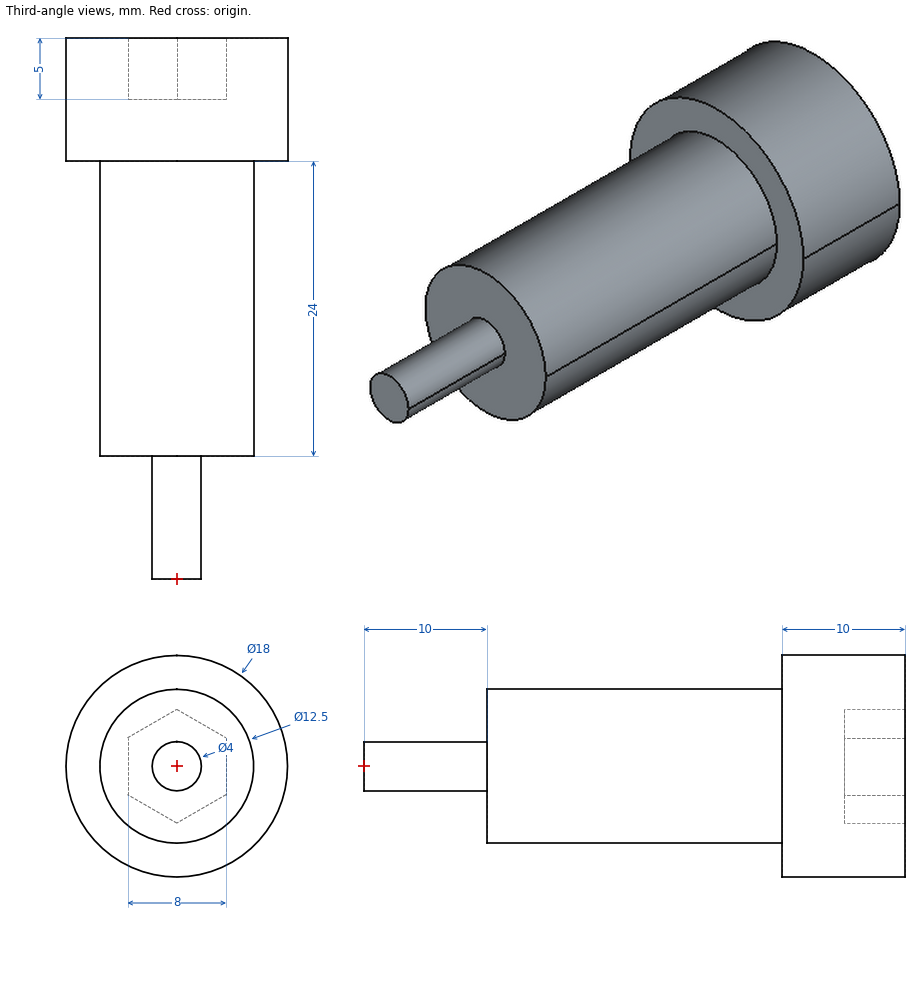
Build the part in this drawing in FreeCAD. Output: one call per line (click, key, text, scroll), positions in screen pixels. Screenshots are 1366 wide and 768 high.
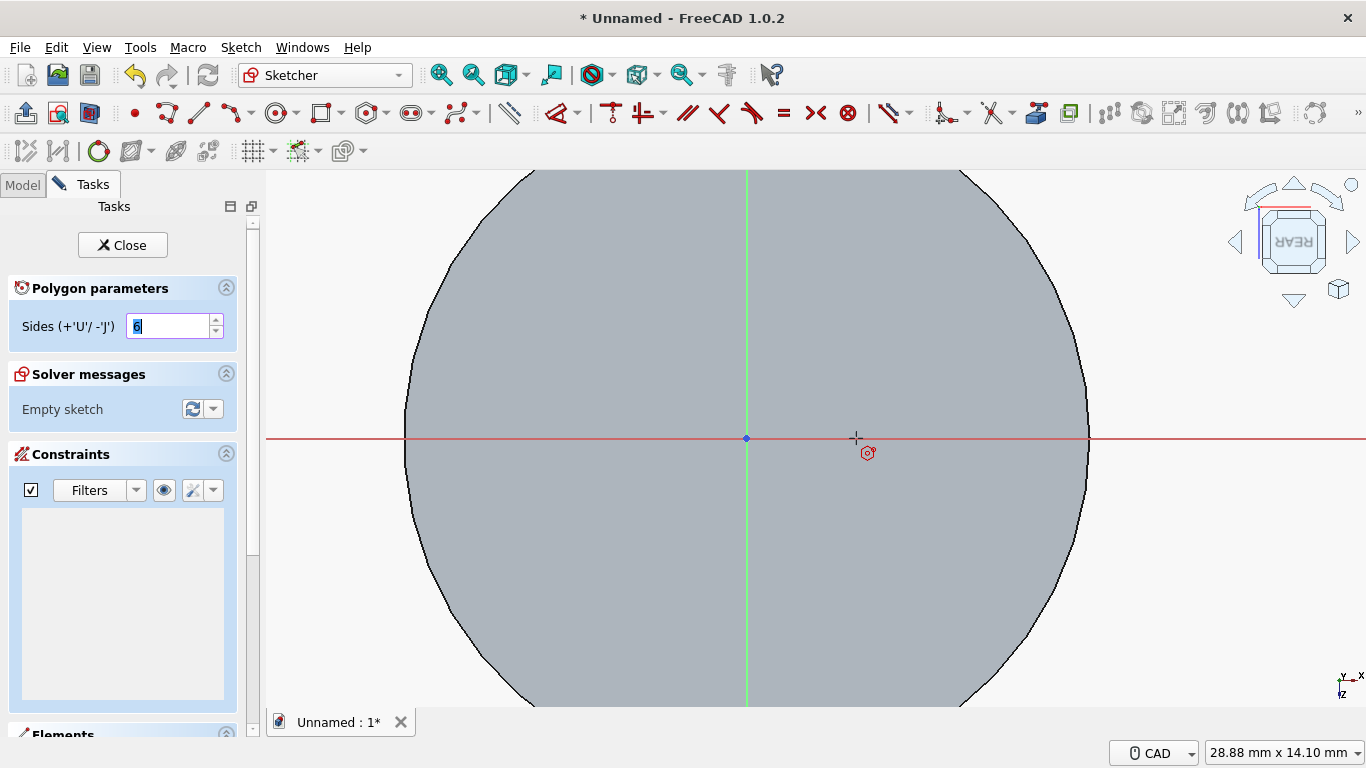
click(747, 438)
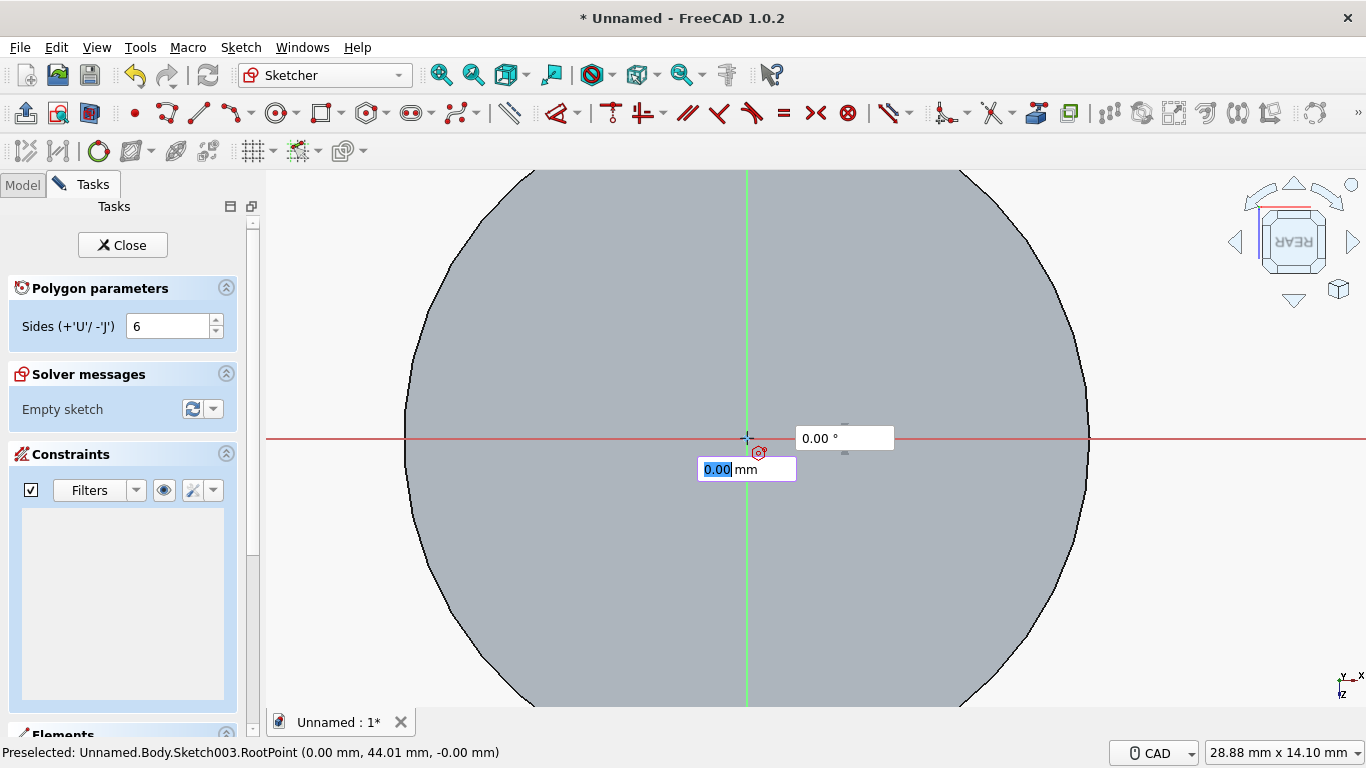
click(747, 263)
right_click(747, 263)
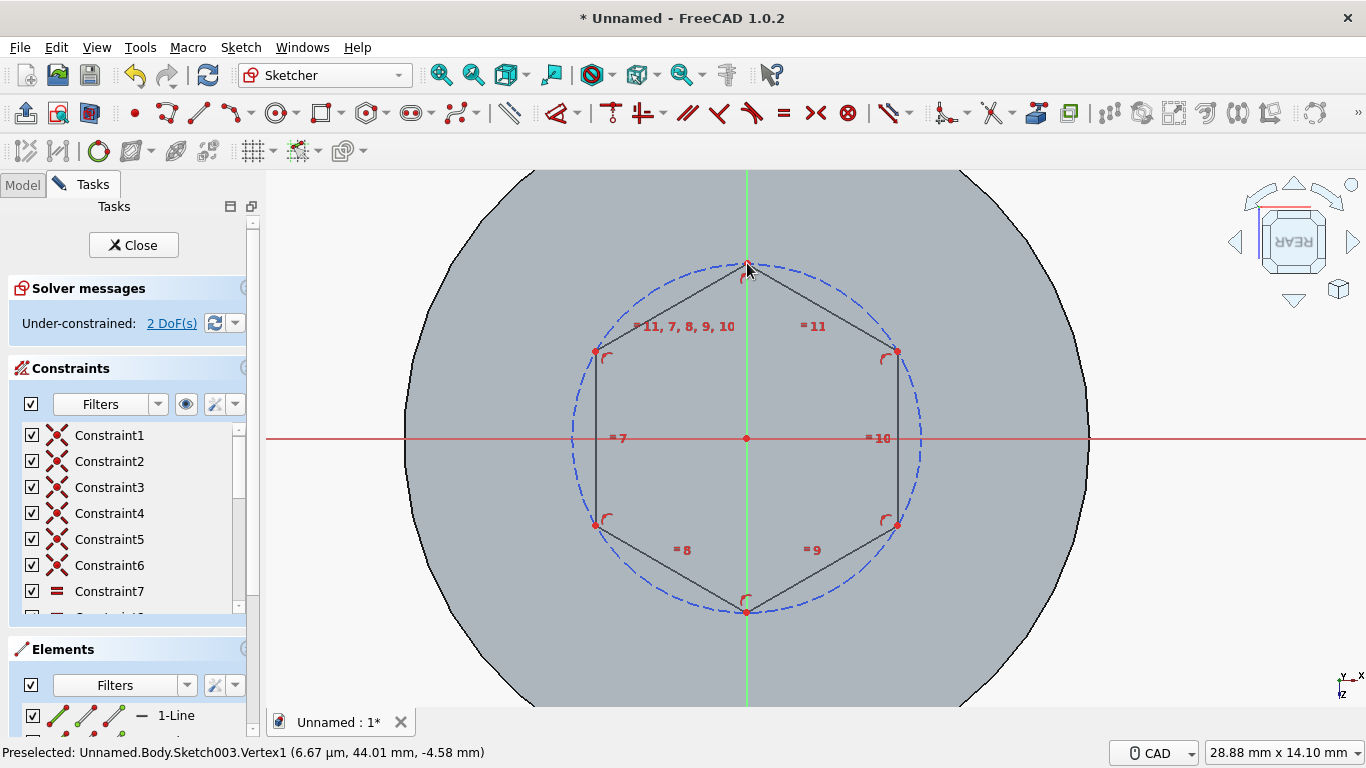
click(596, 403)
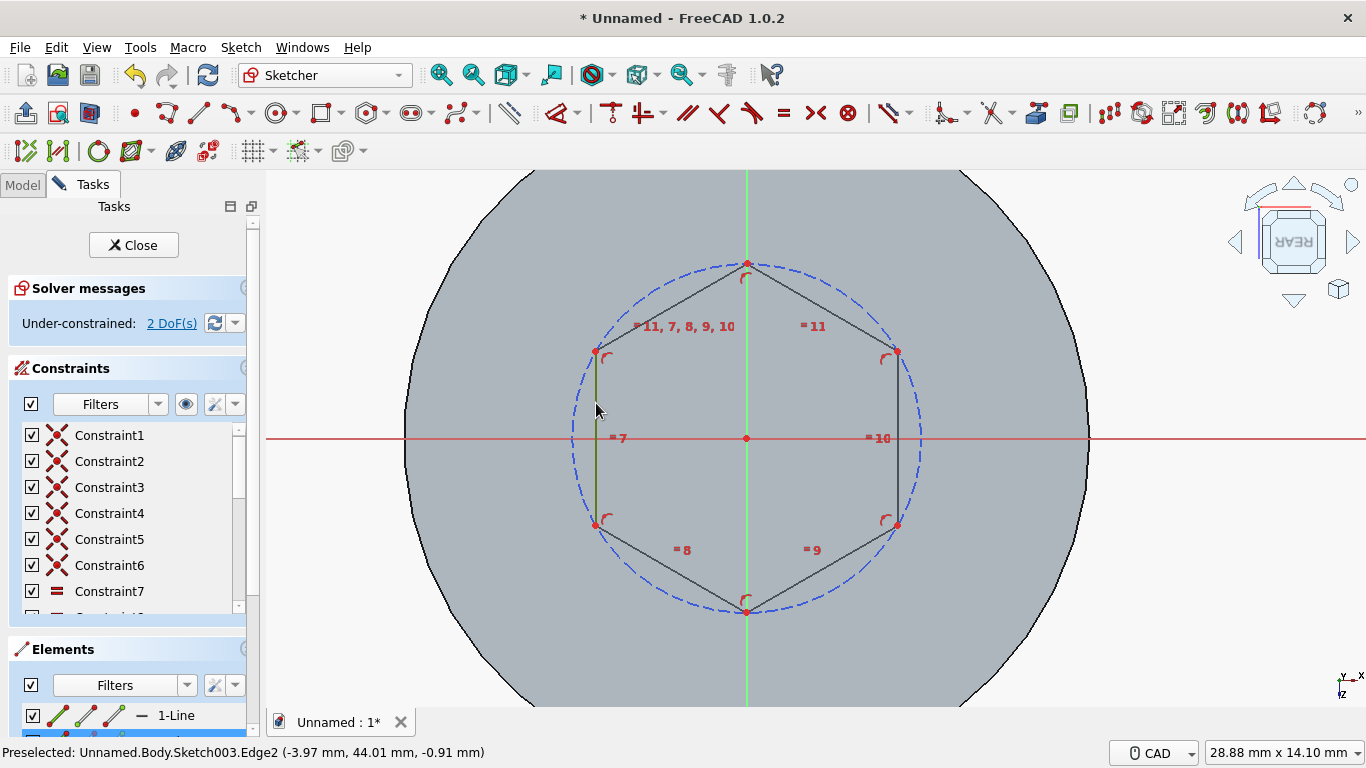
key(v)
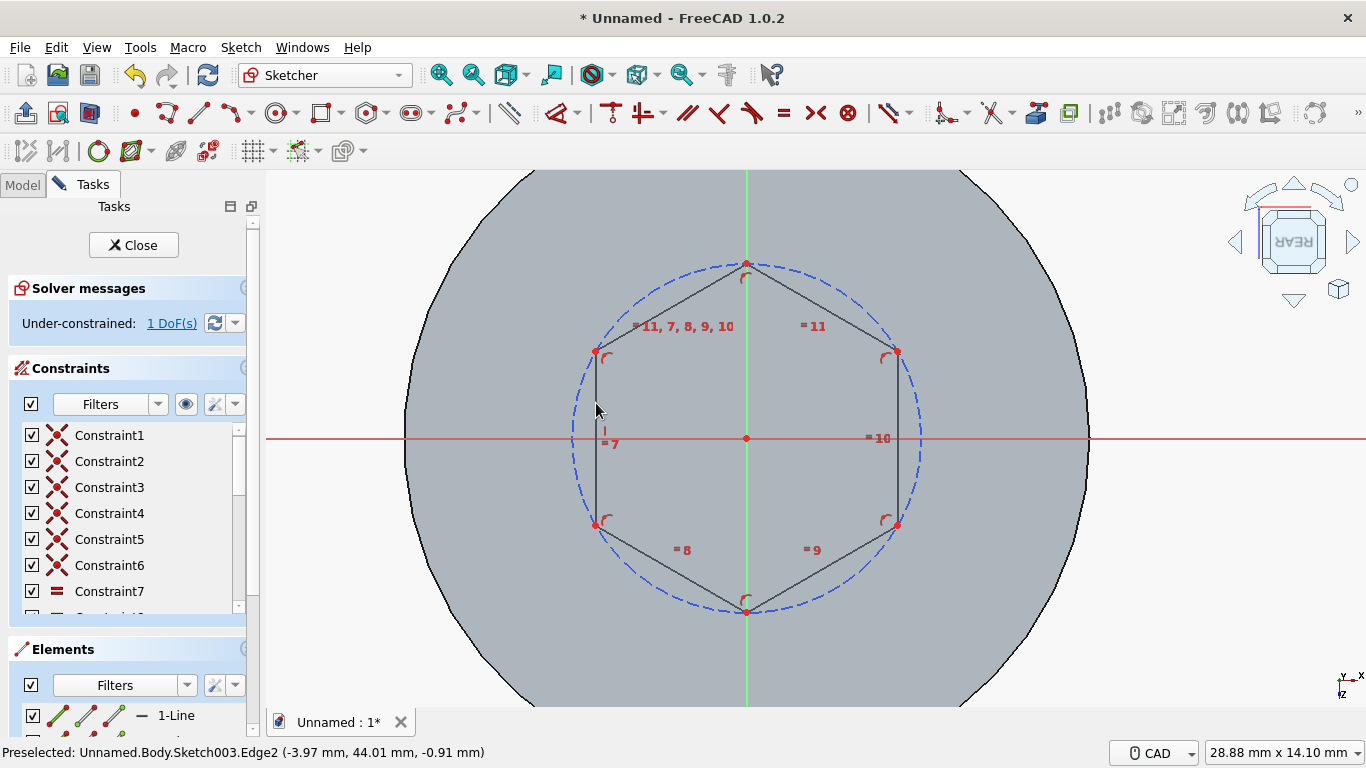
key(d)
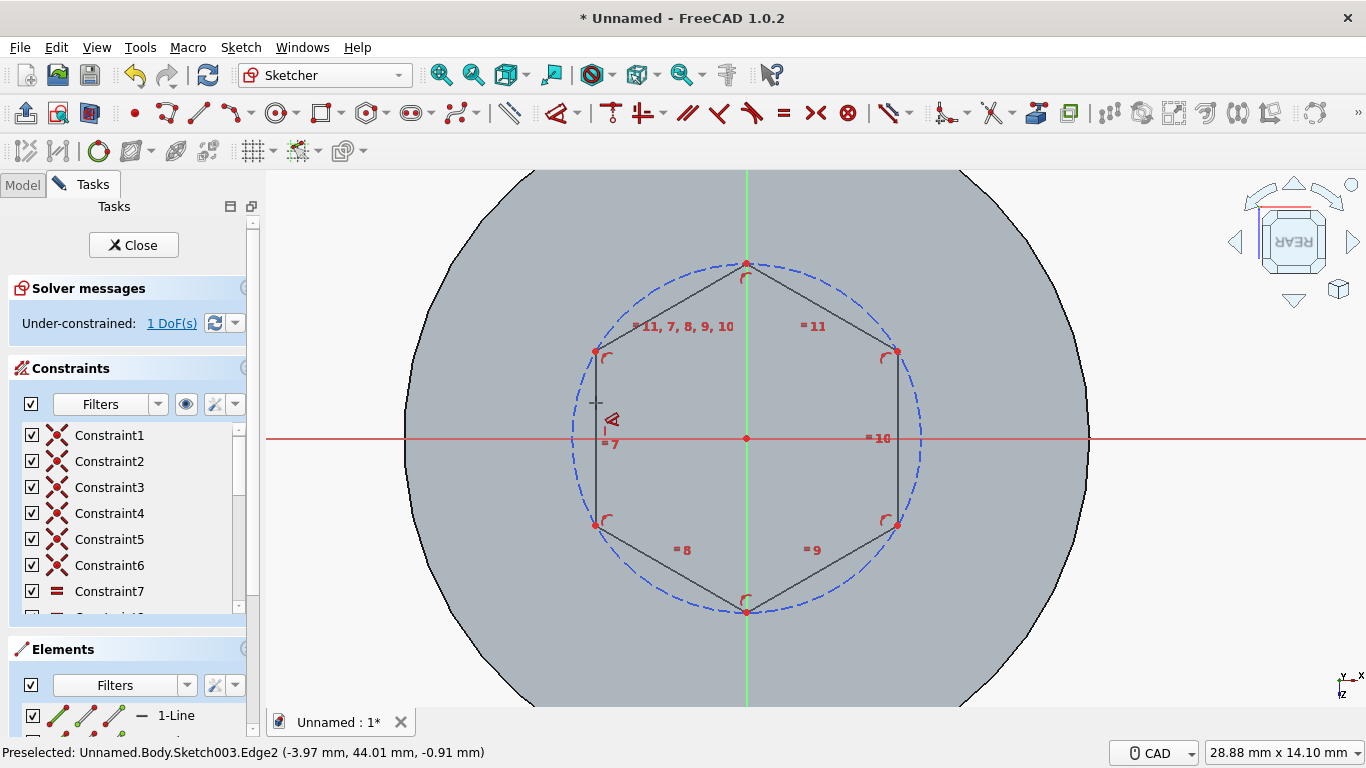
click(596, 351)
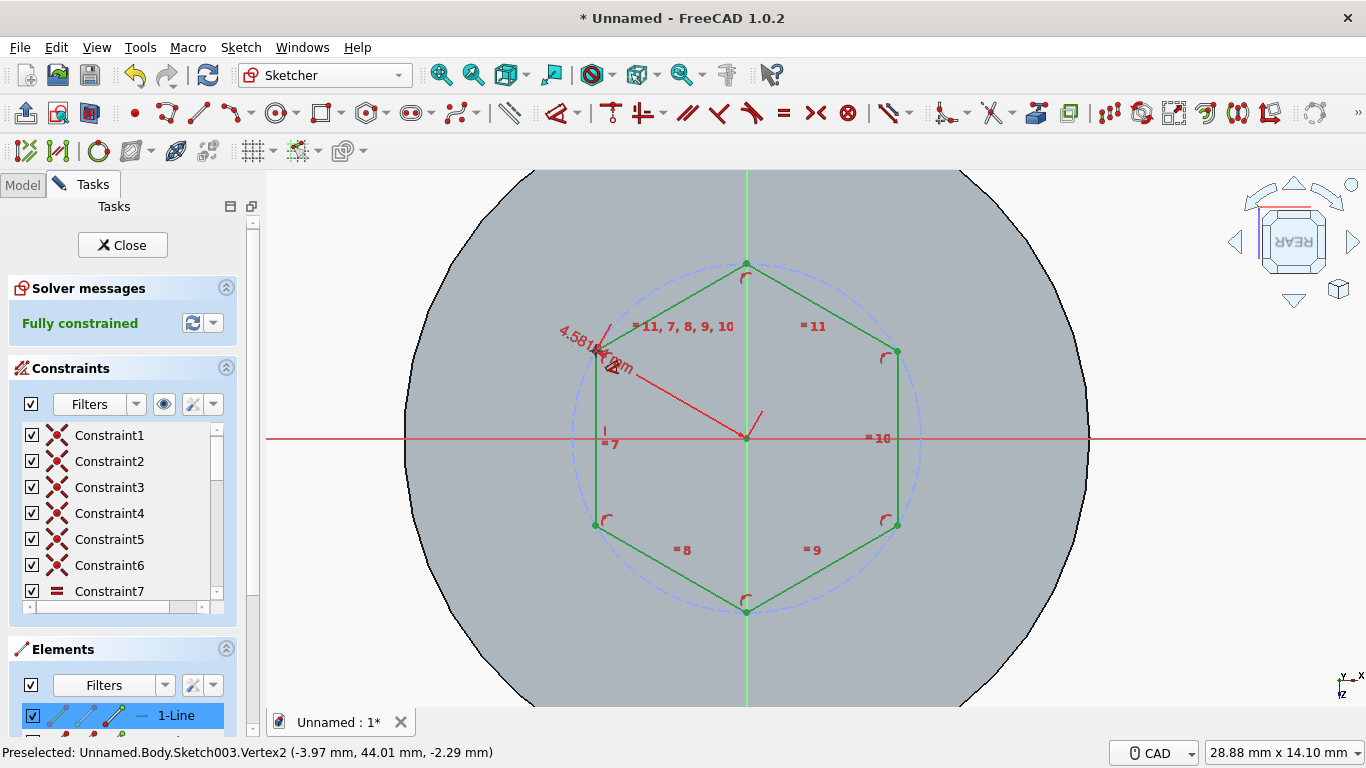
click(898, 526)
click(641, 269)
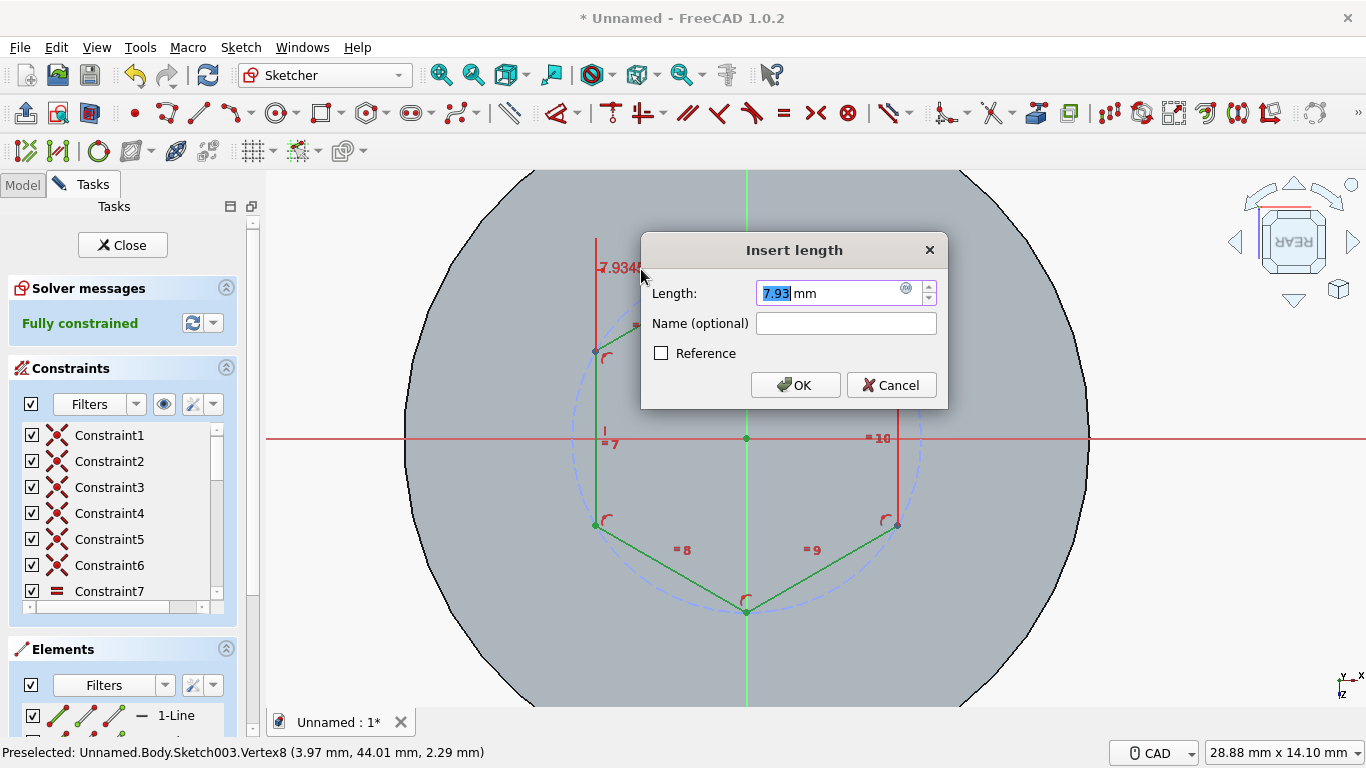
text(8)
key(Return)
key(Escape)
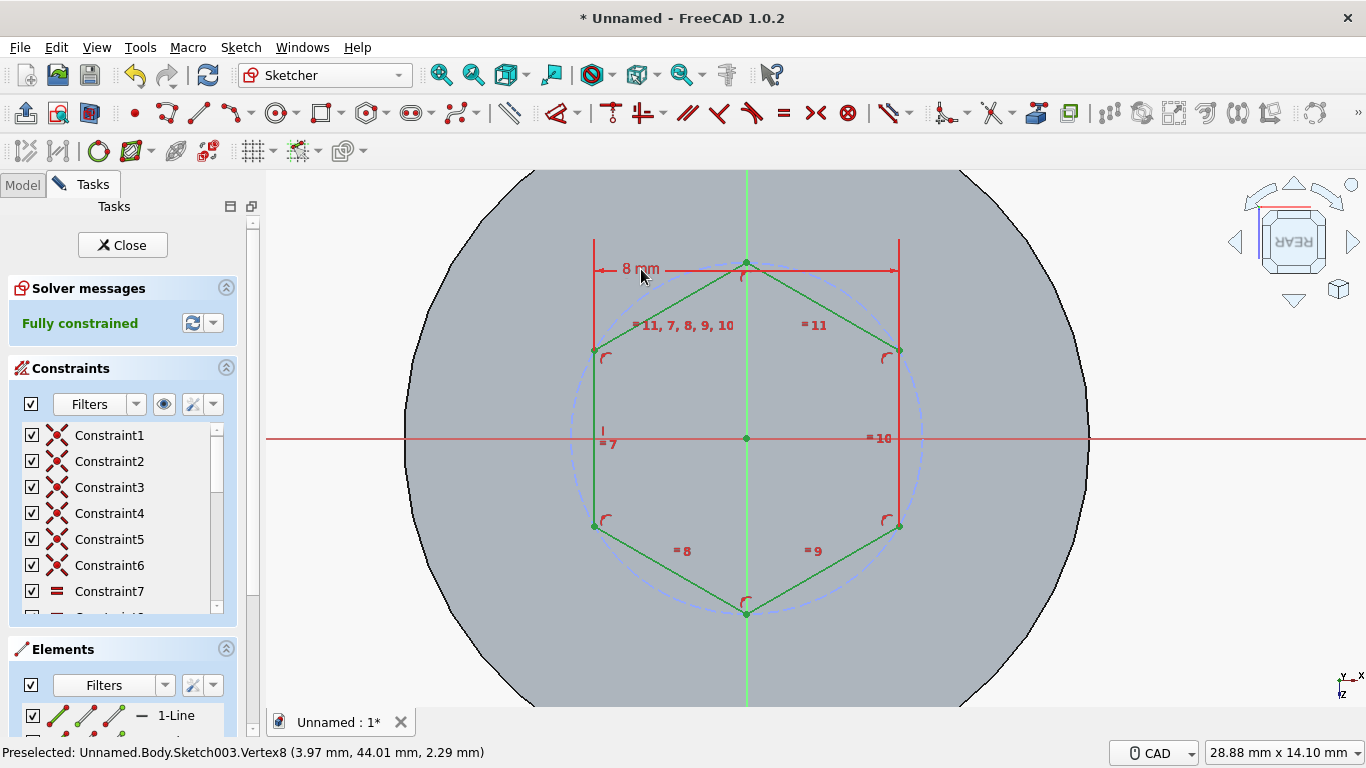
click(123, 245)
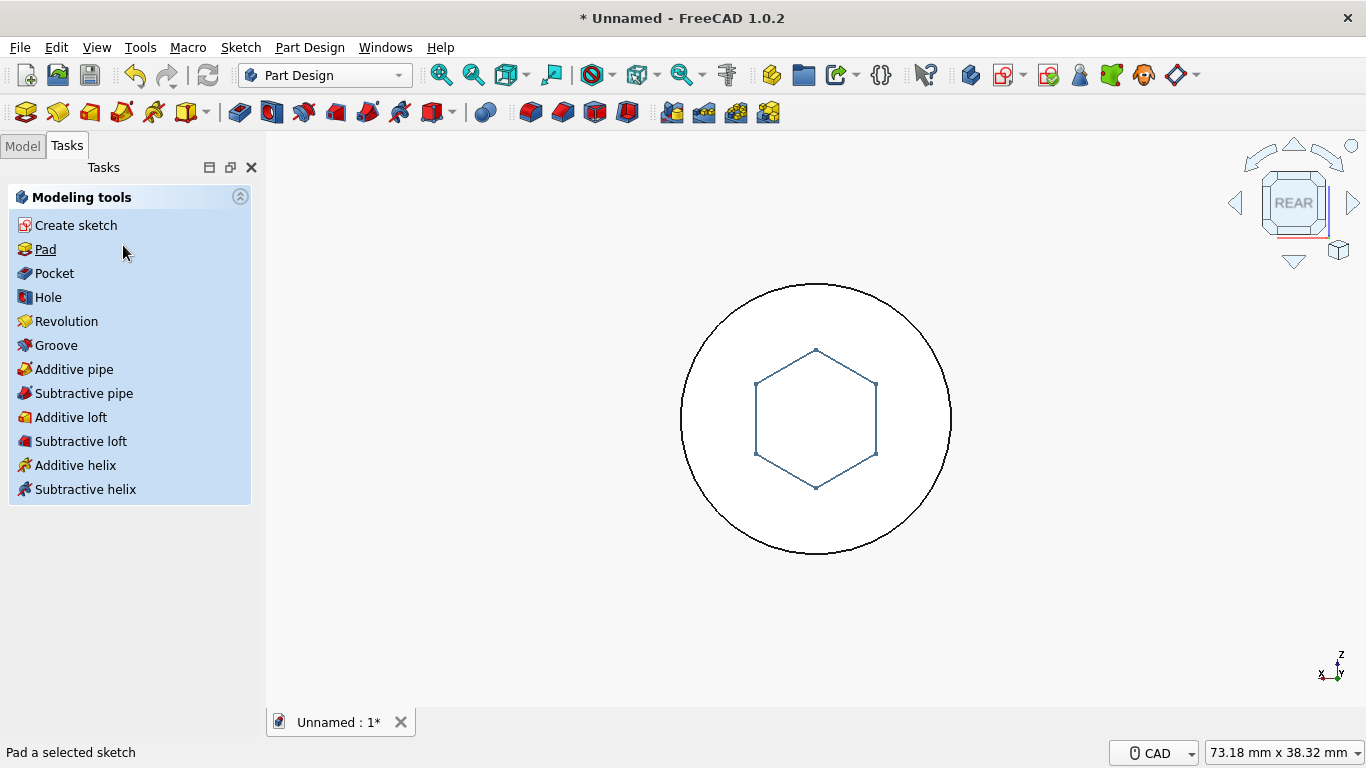
click(240, 112)